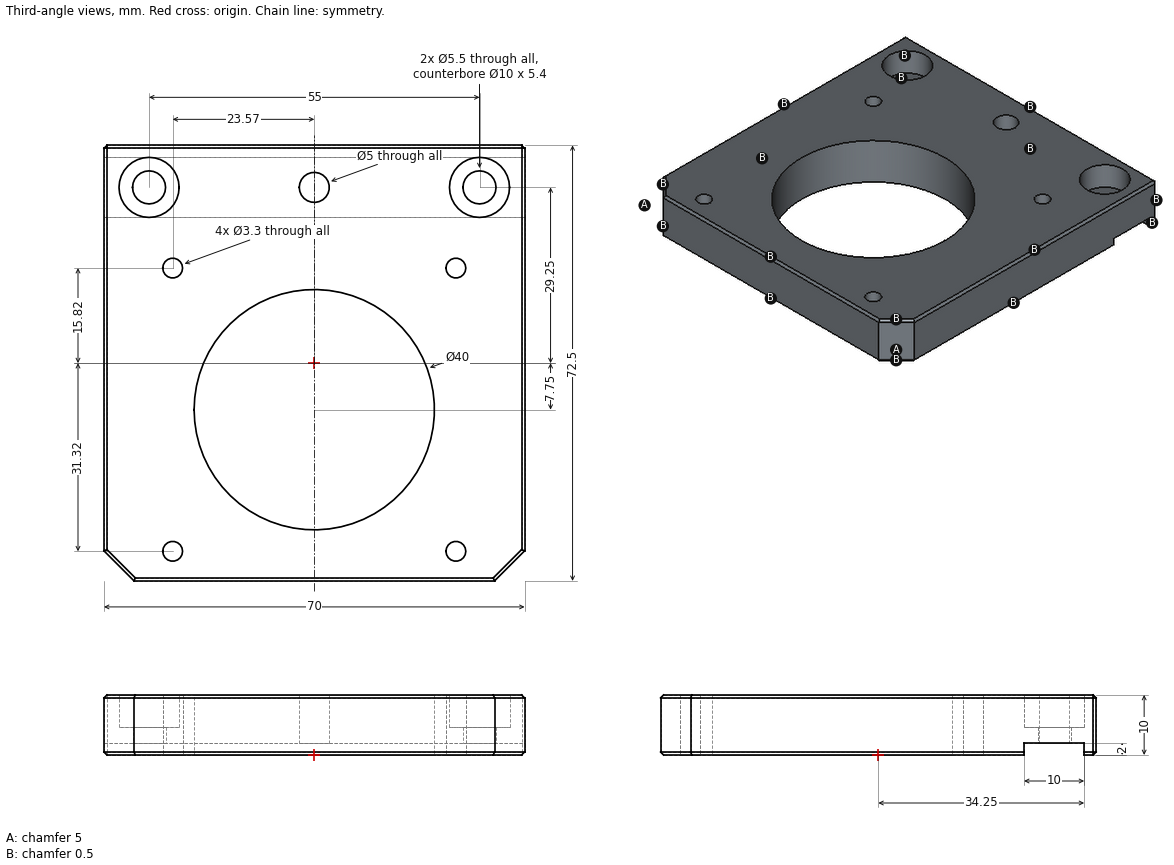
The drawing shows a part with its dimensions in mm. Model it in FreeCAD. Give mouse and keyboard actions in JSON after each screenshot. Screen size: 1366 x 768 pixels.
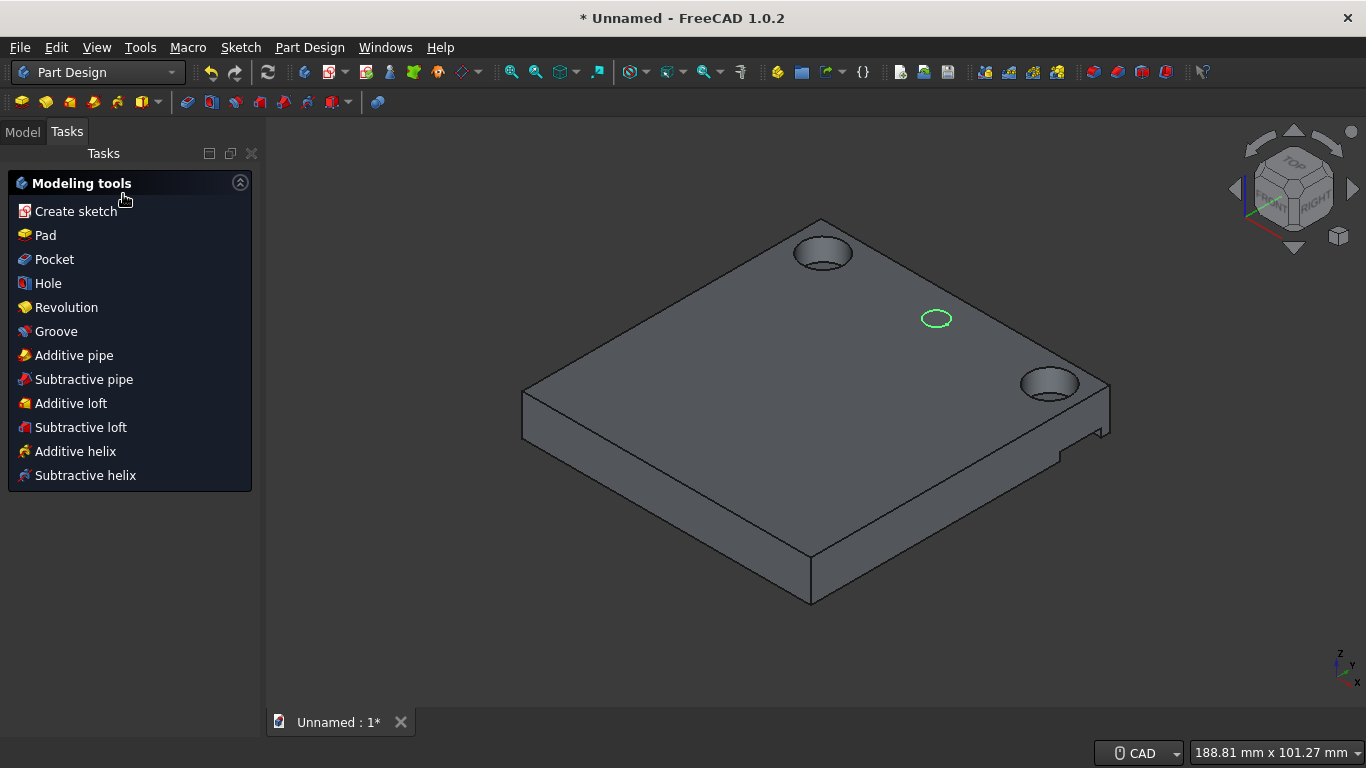
{"action": "left_click", "coordinate": [212, 102]}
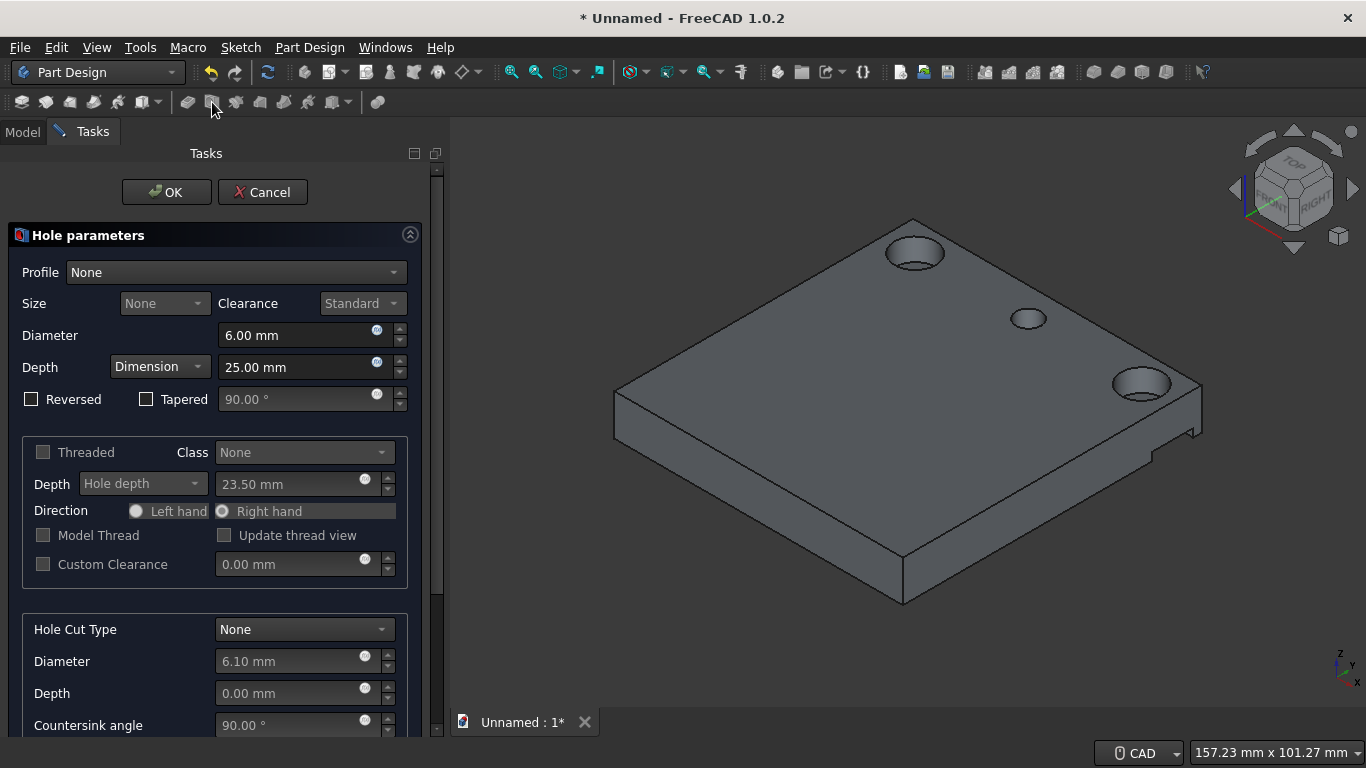
{"action": "triple_click", "coordinate": [305, 335]}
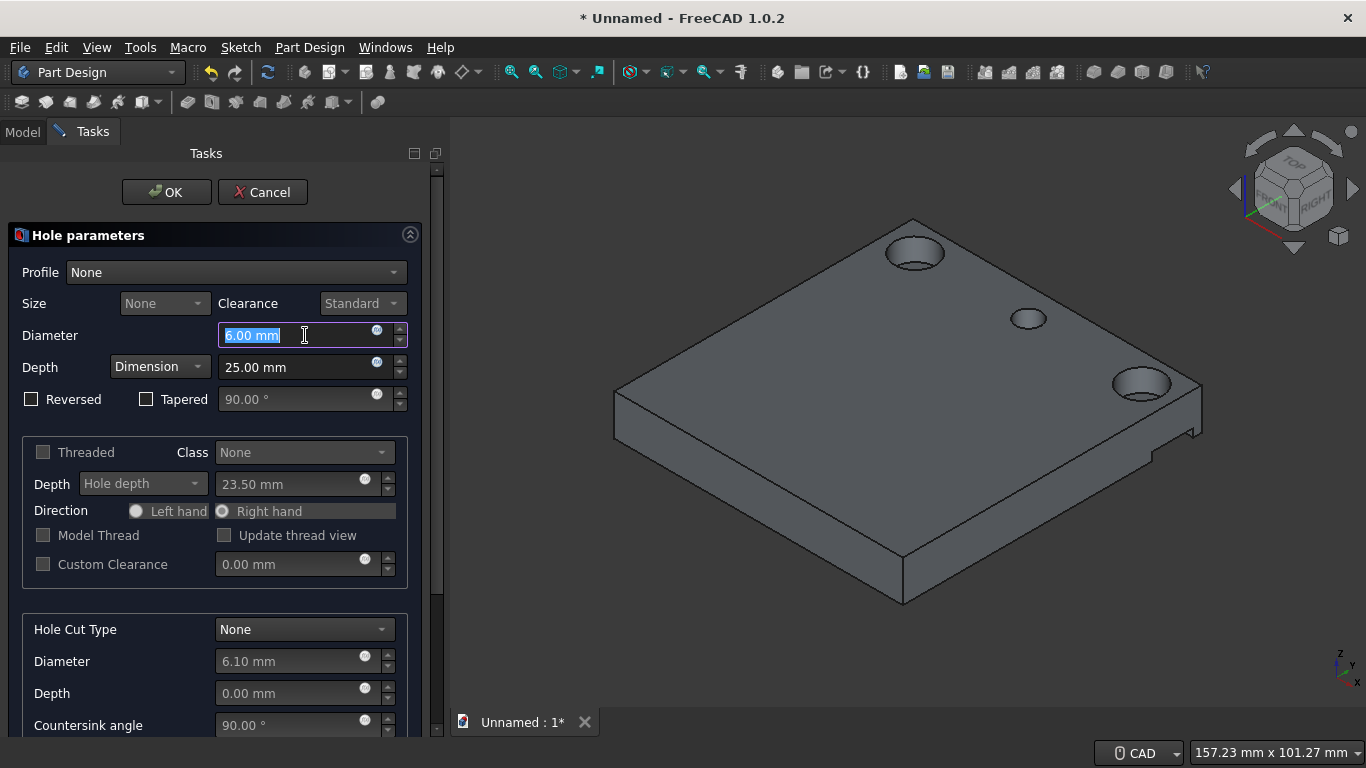
{"action": "type", "text": "5"}
{"action": "key", "text": "Tab"}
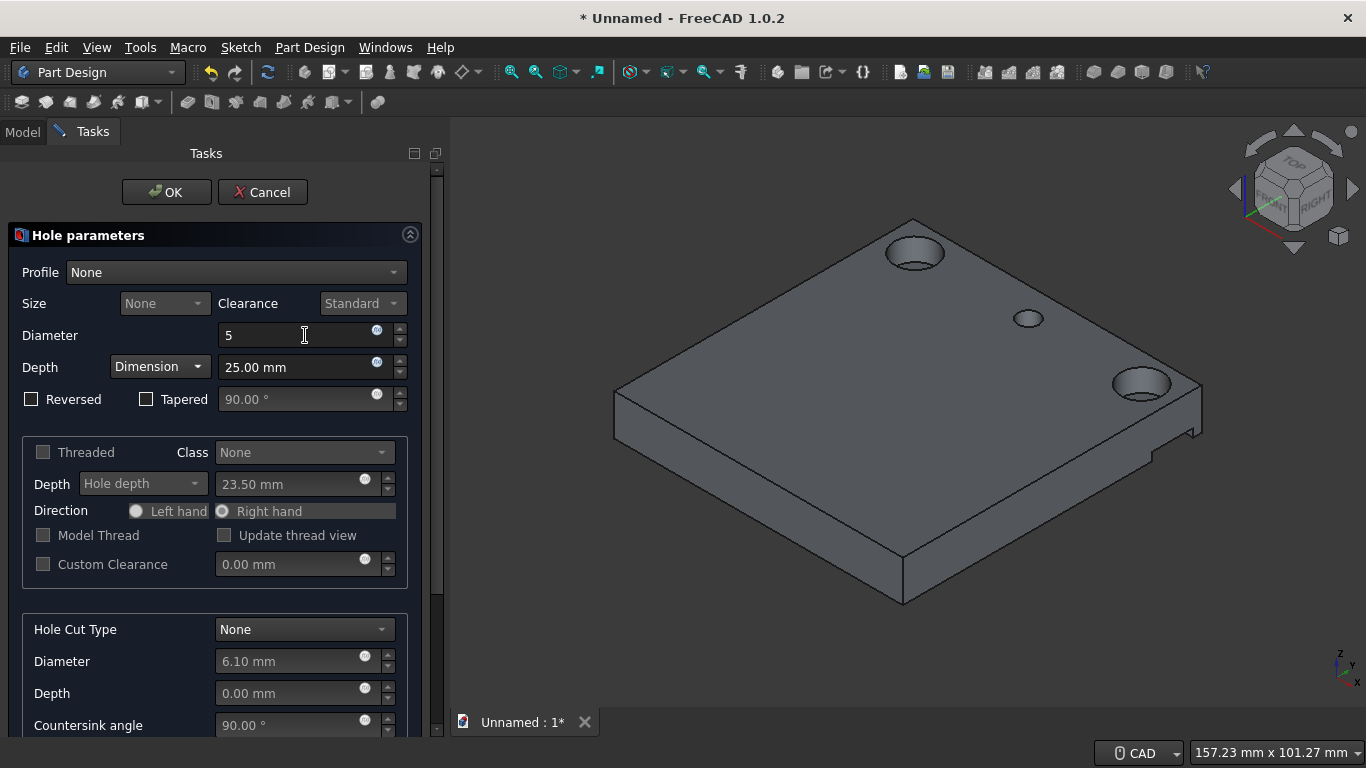
{"action": "left_click", "coordinate": [161, 366]}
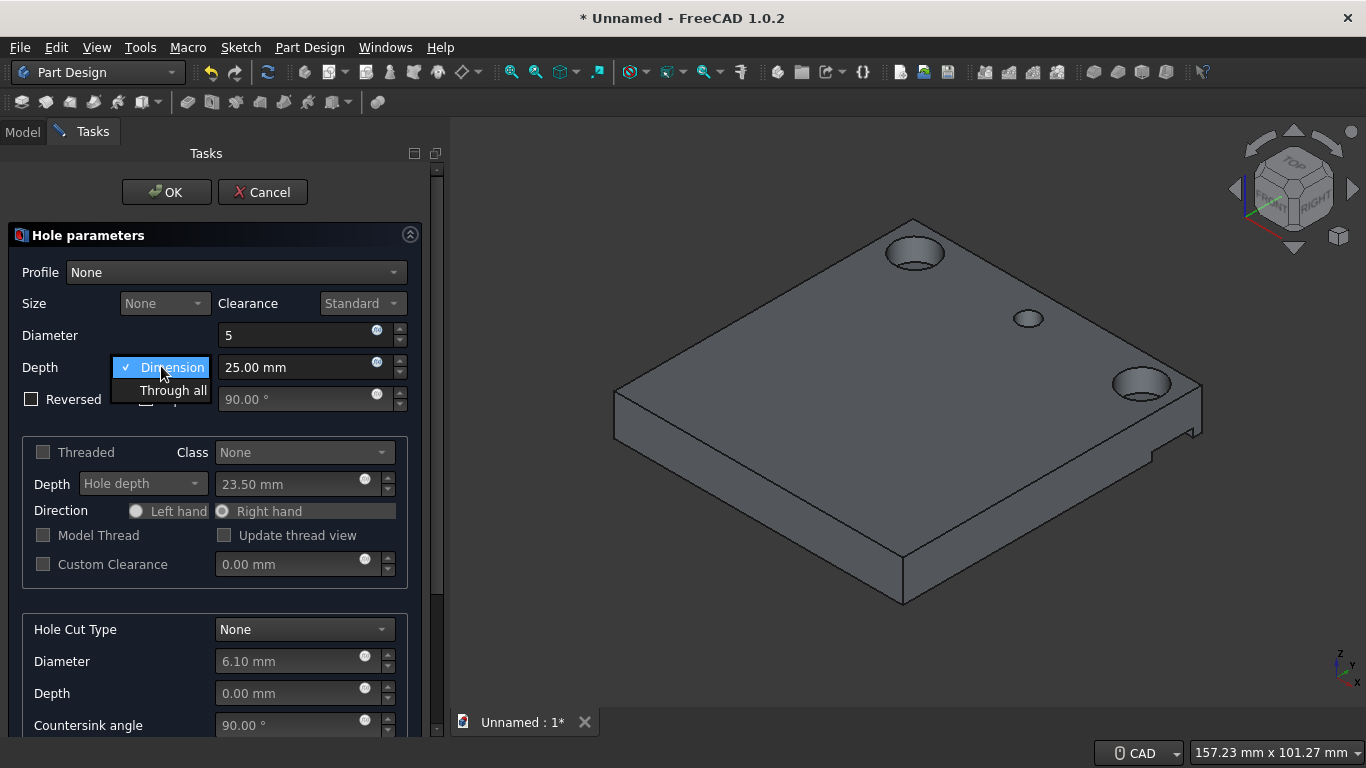
{"action": "left_click", "coordinate": [160, 390]}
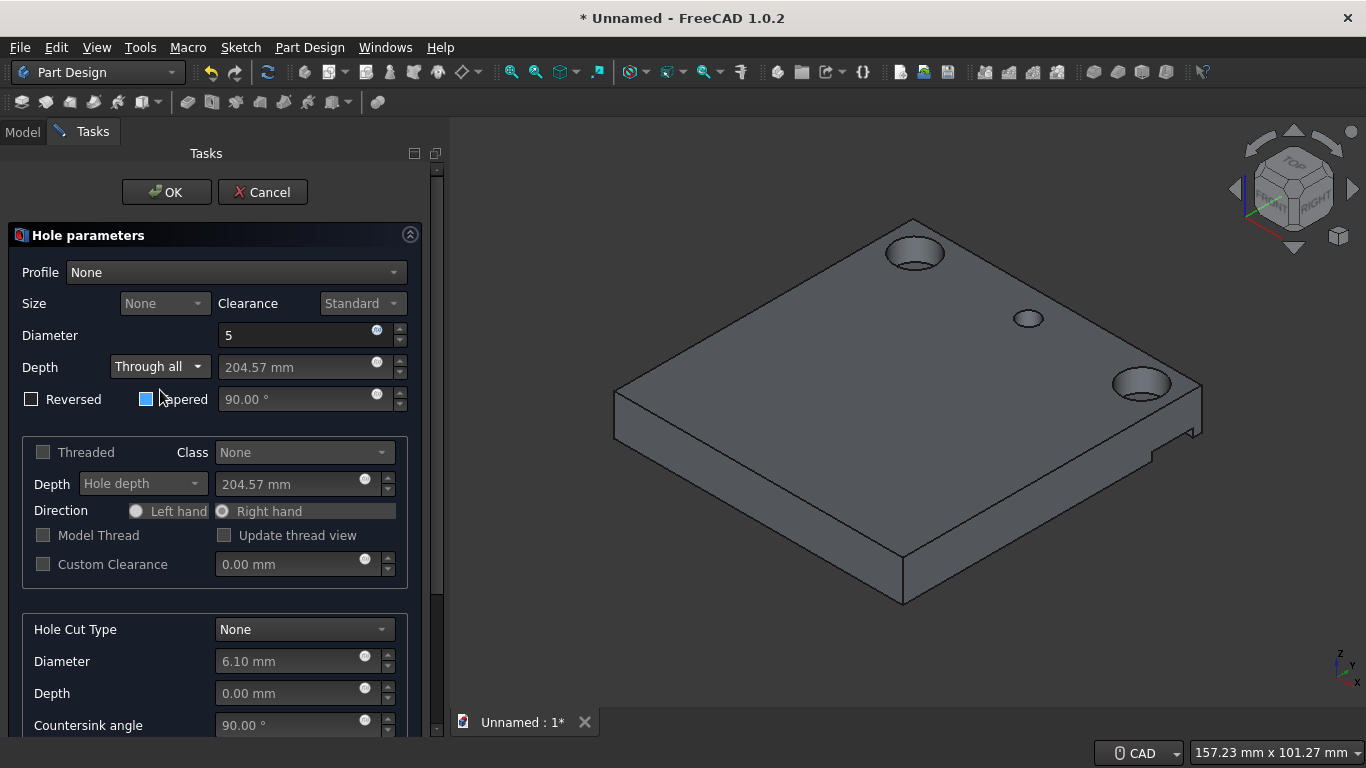
{"action": "left_click", "coordinate": [167, 192]}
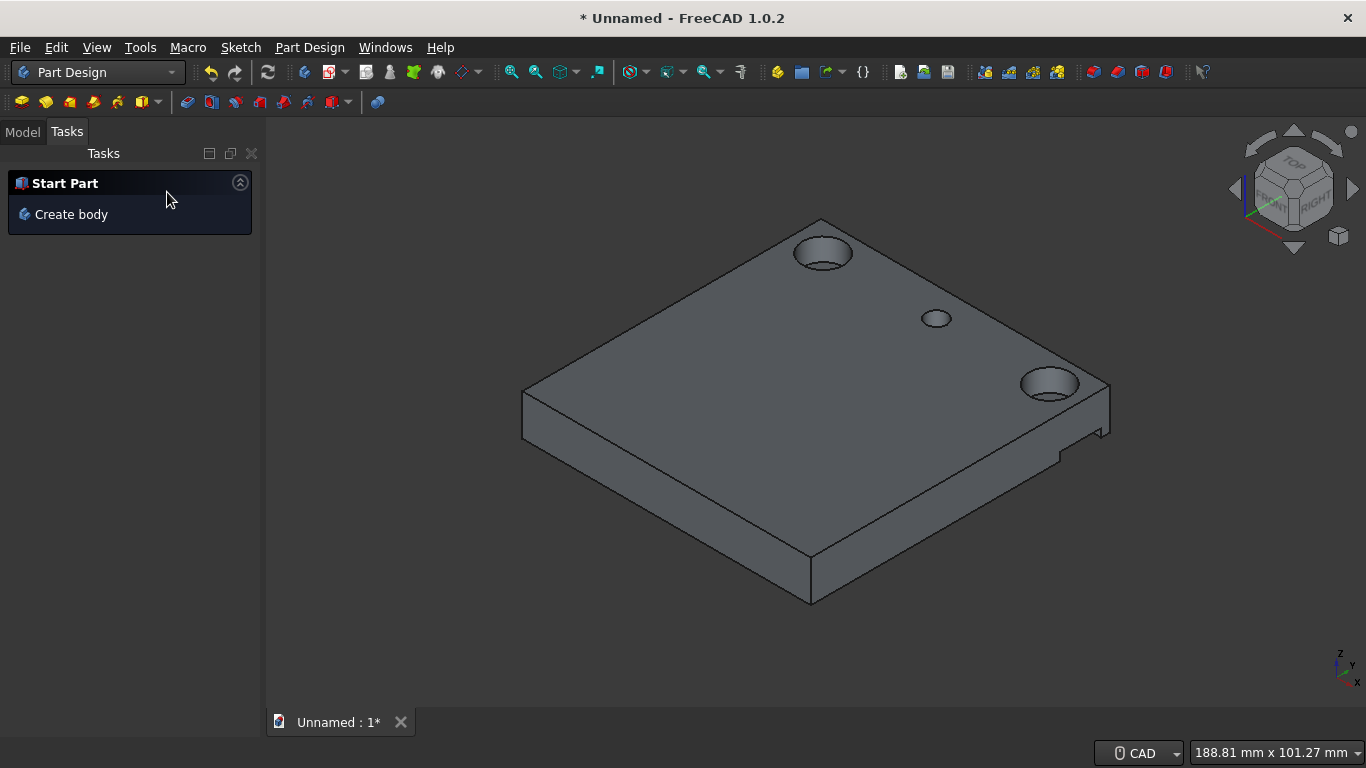
{"action": "left_click", "coordinate": [816, 387]}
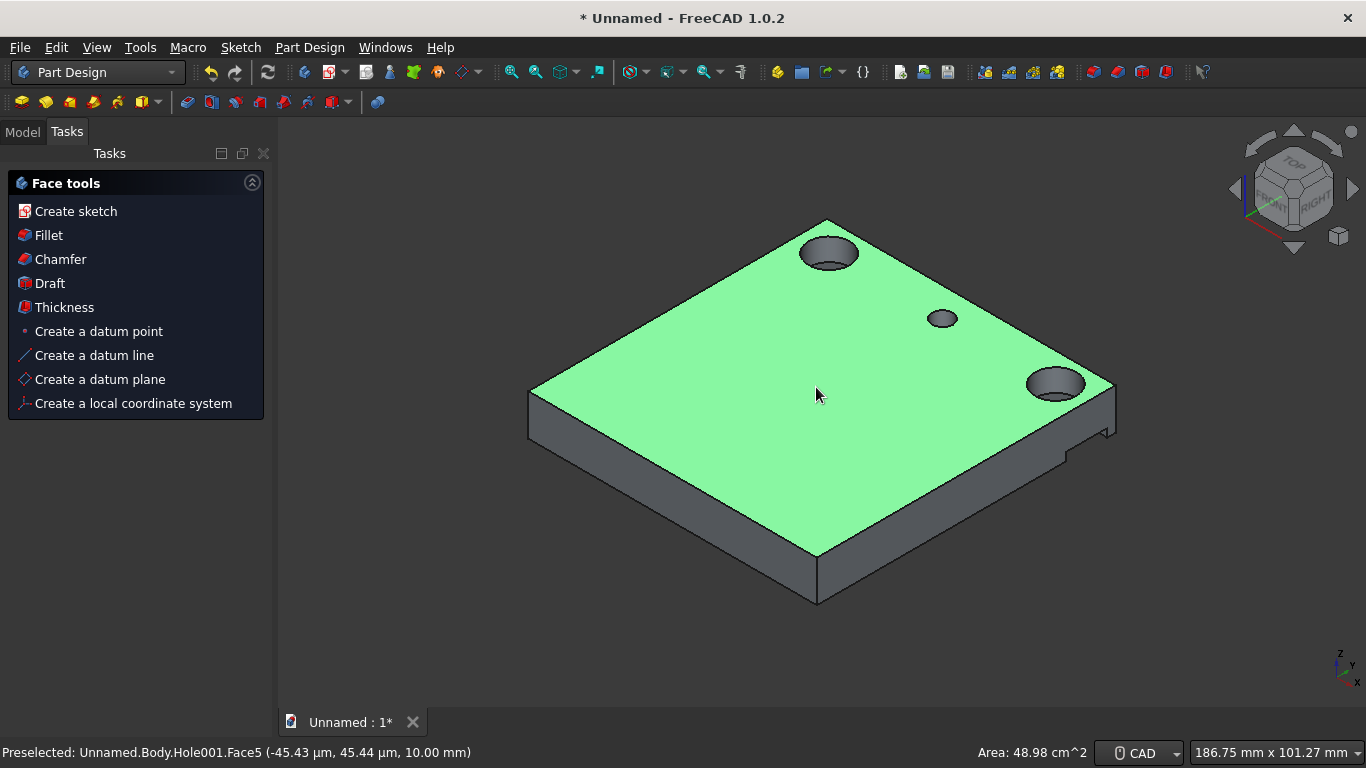
{"action": "left_click", "coordinate": [330, 72]}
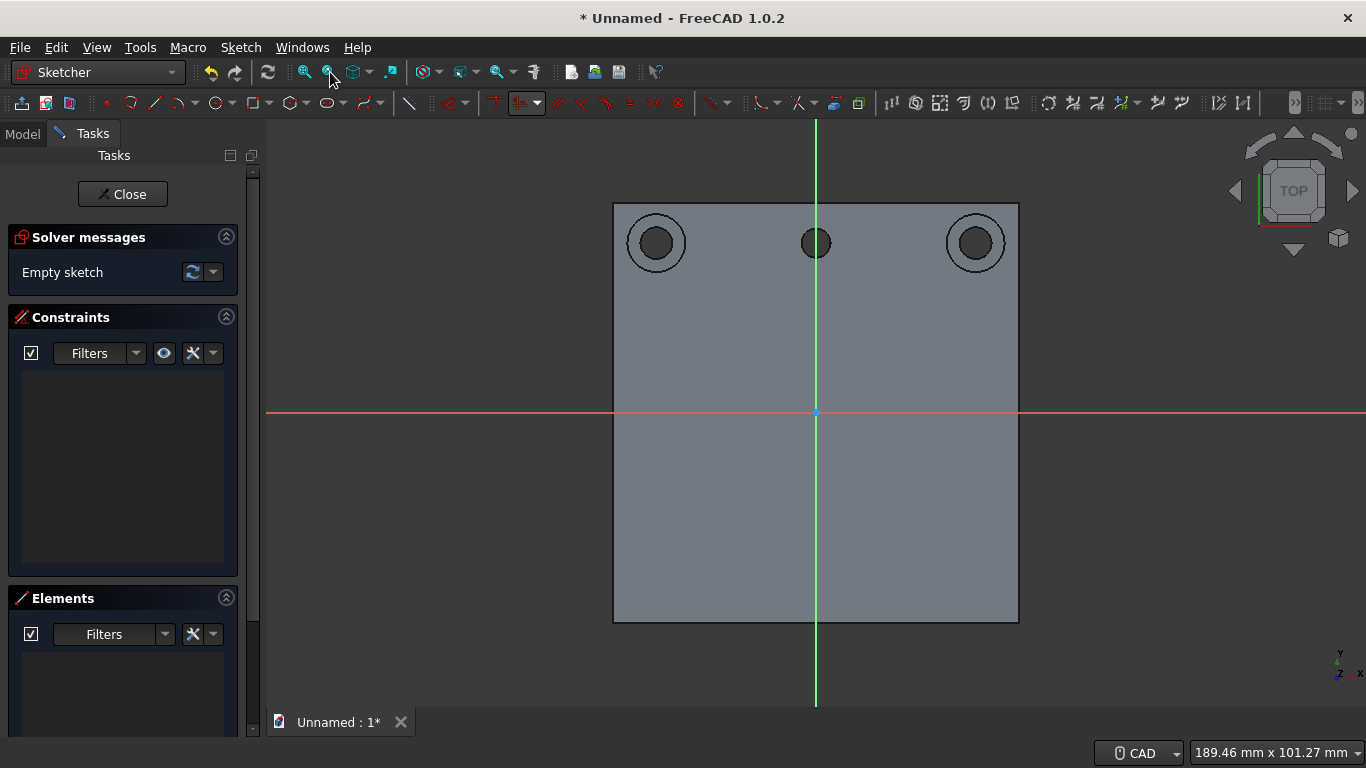
{"action": "left_click", "coordinate": [216, 104]}